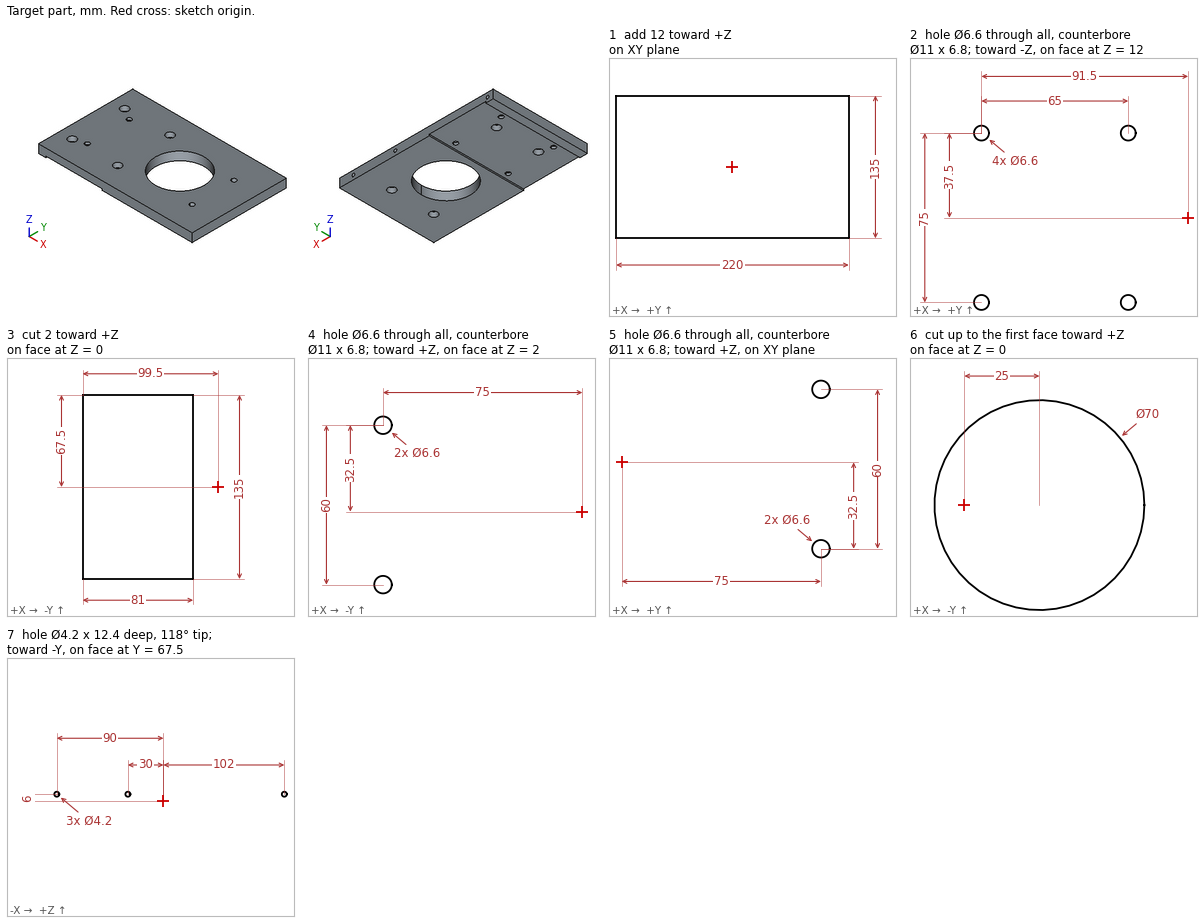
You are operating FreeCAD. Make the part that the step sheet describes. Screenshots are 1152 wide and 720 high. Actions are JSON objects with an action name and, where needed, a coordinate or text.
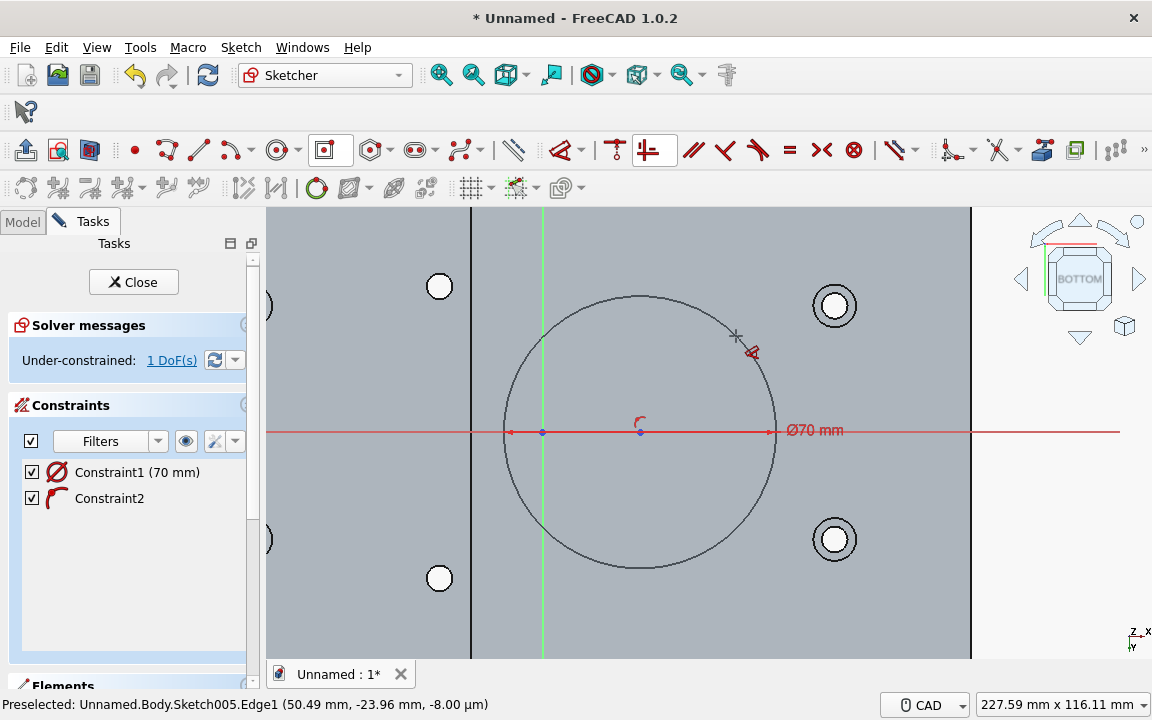
{"action": "left_click", "coordinate": [640, 432]}
{"action": "left_click", "coordinate": [591, 466]}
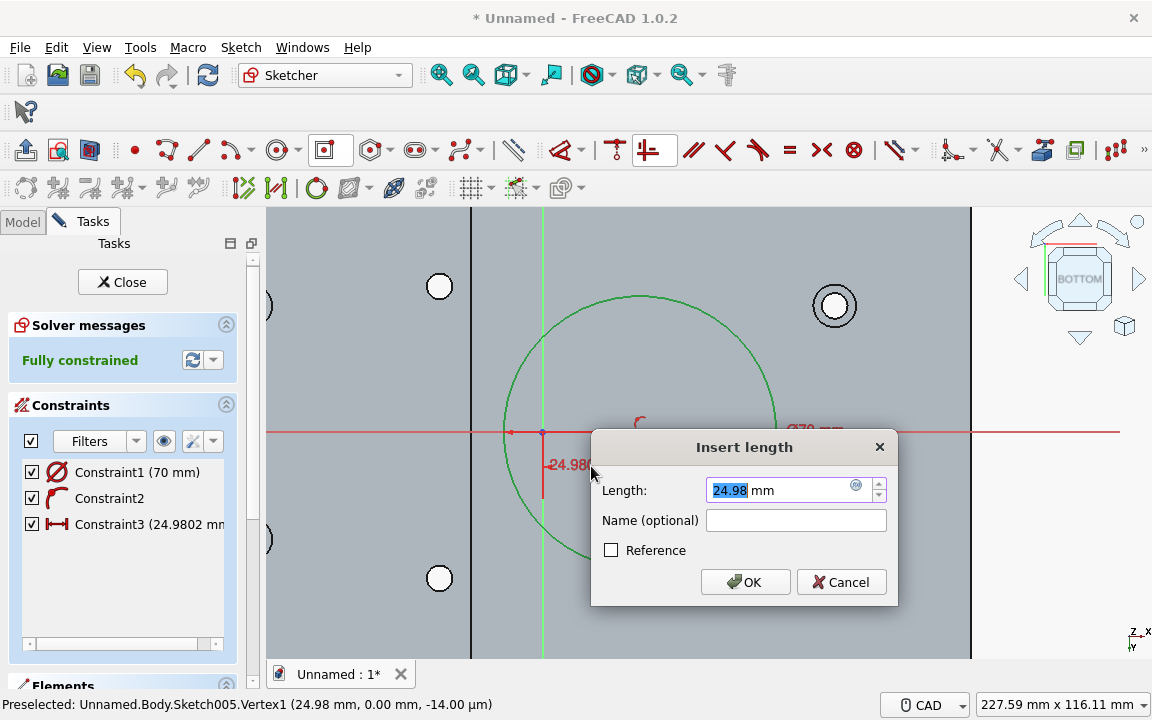
{"action": "type", "text": "25"}
{"action": "key", "text": "Return"}
{"action": "key", "text": "Escape"}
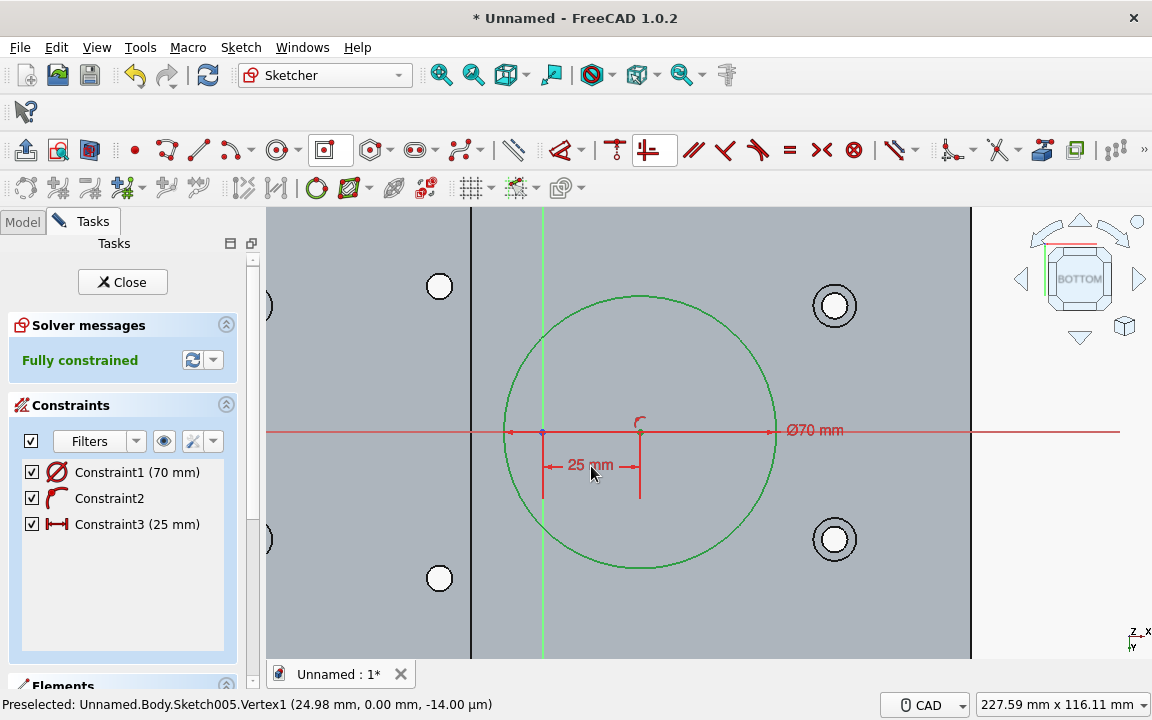
{"action": "left_click", "coordinate": [123, 282]}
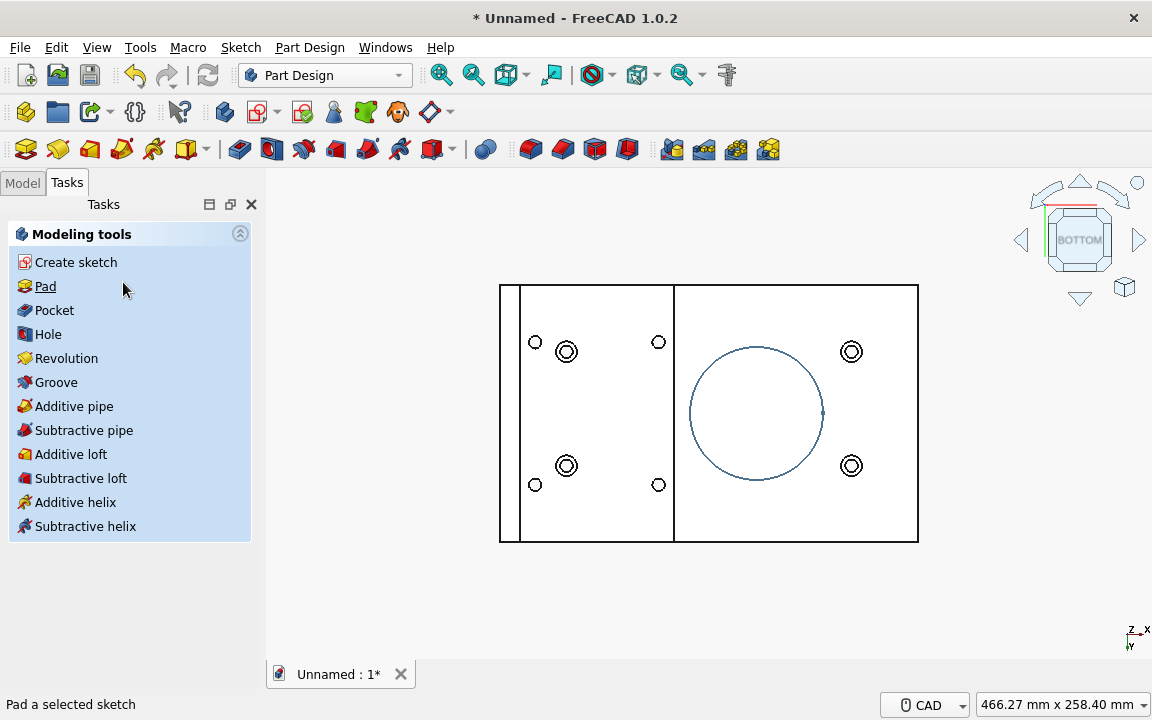
{"action": "left_click", "coordinate": [240, 150]}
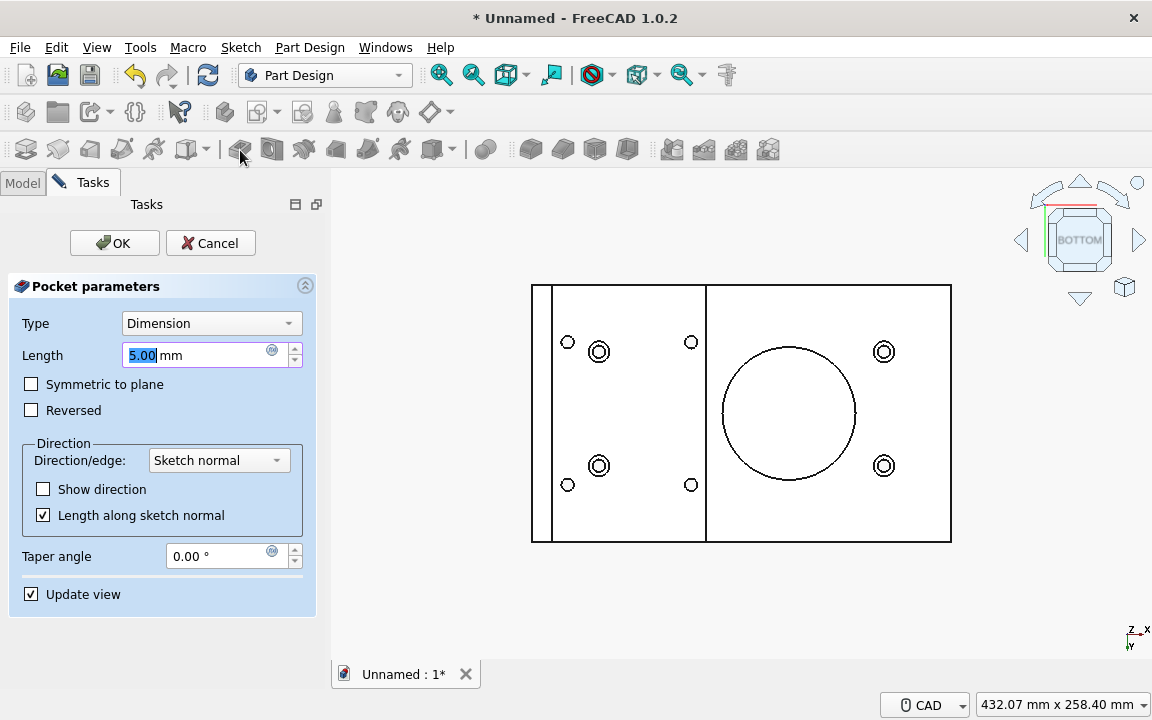
{"action": "left_click", "coordinate": [212, 324]}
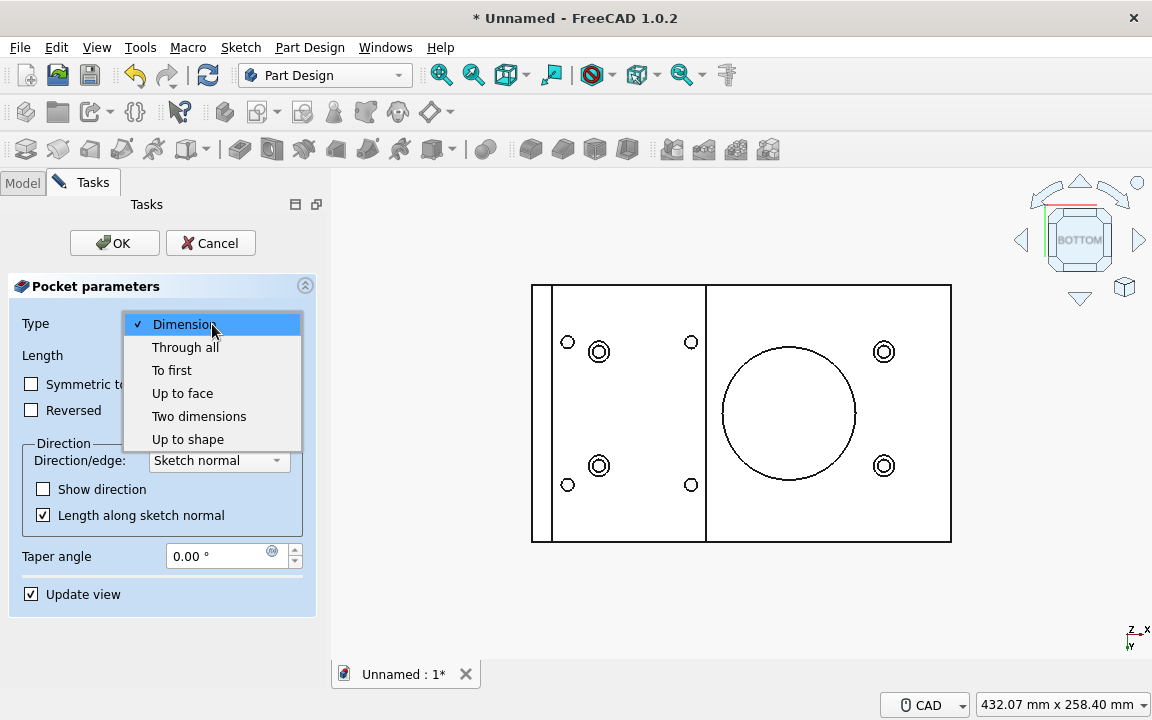
{"action": "left_click", "coordinate": [212, 370]}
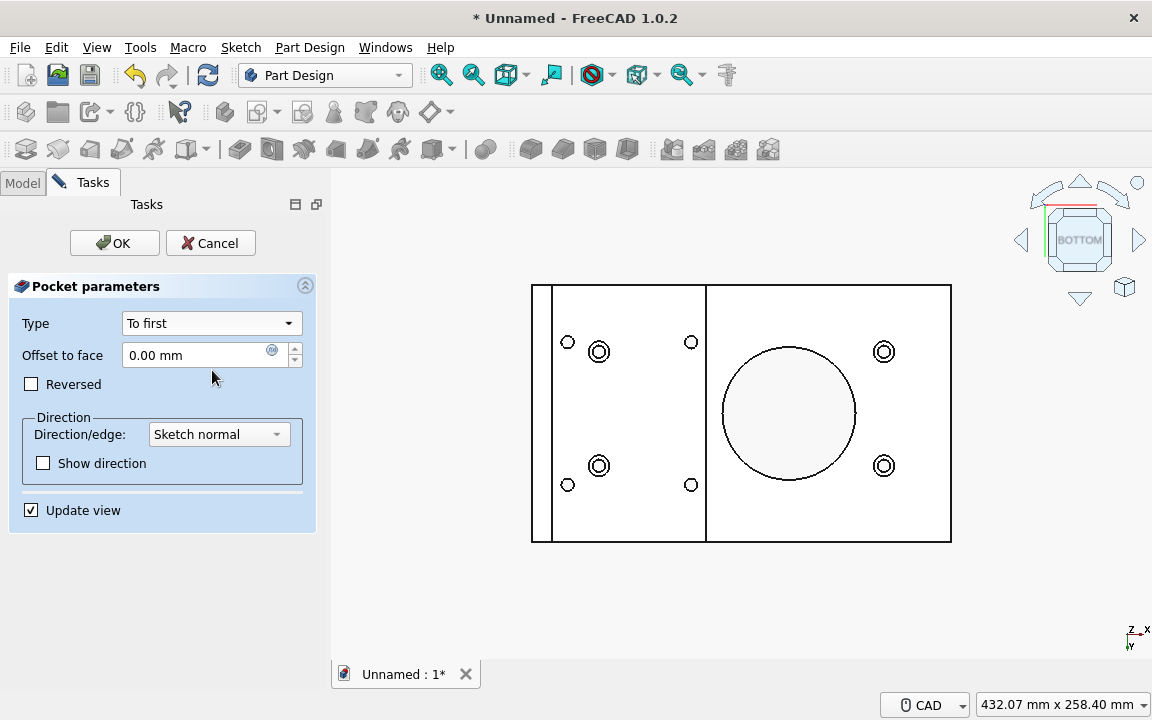
{"action": "left_click", "coordinate": [115, 243]}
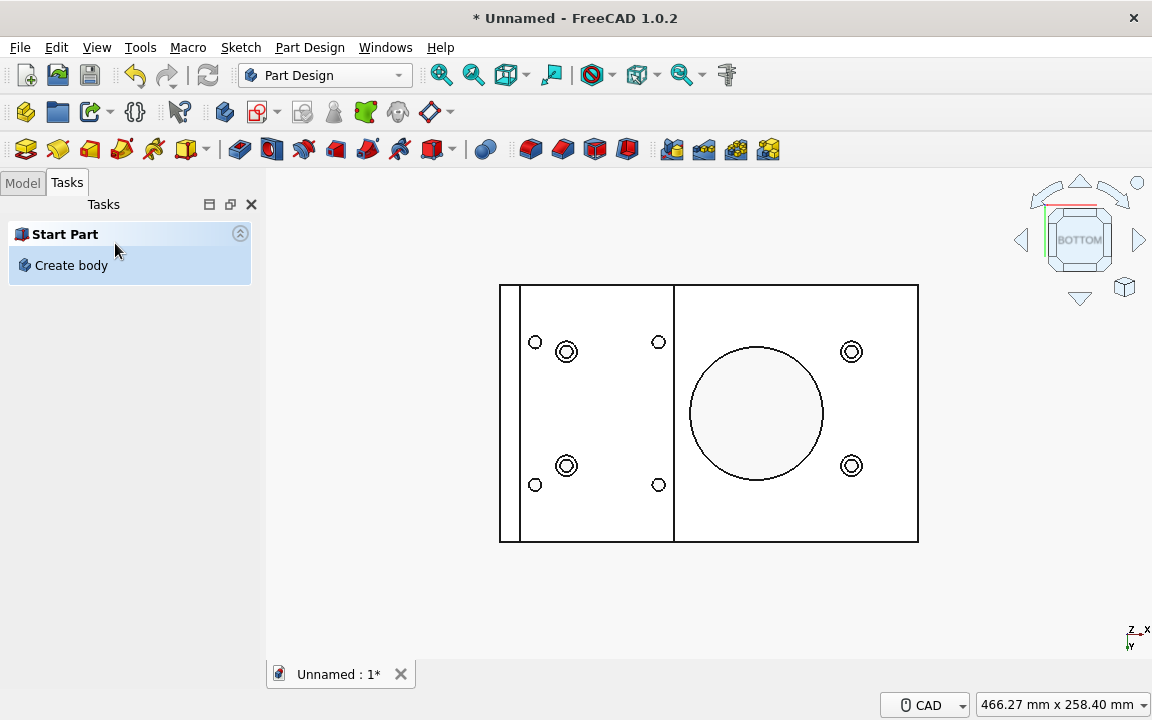
{"action": "key", "text": "4"}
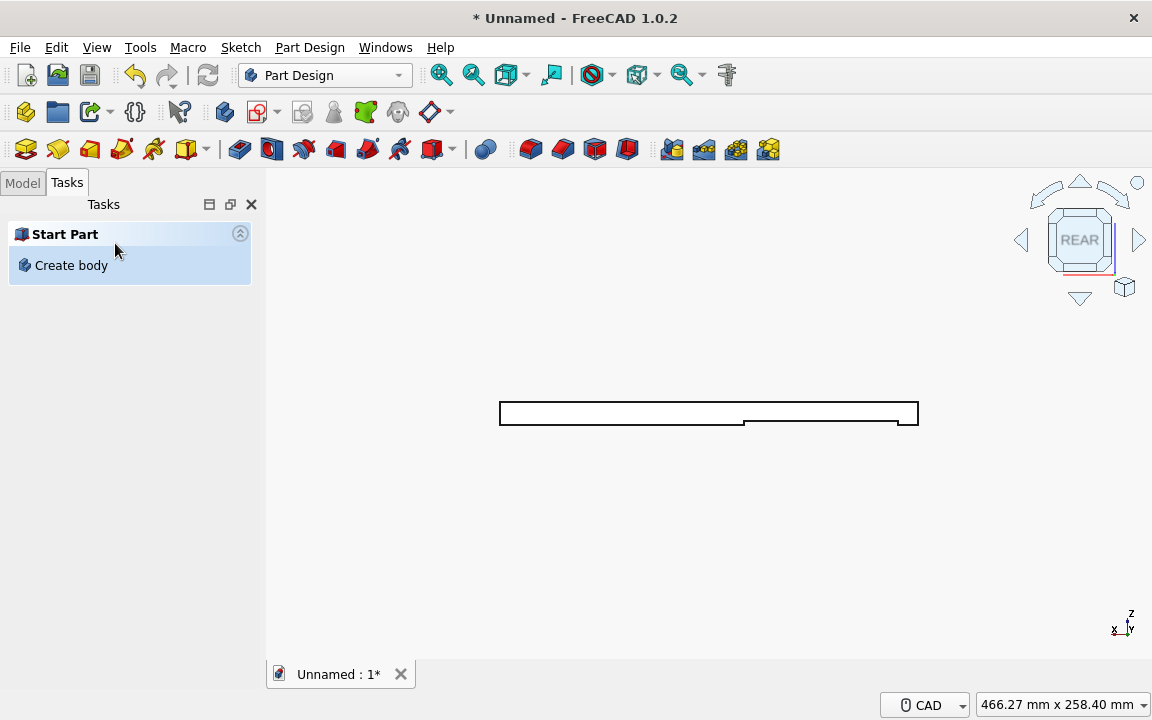
{"action": "left_click", "coordinate": [530, 412]}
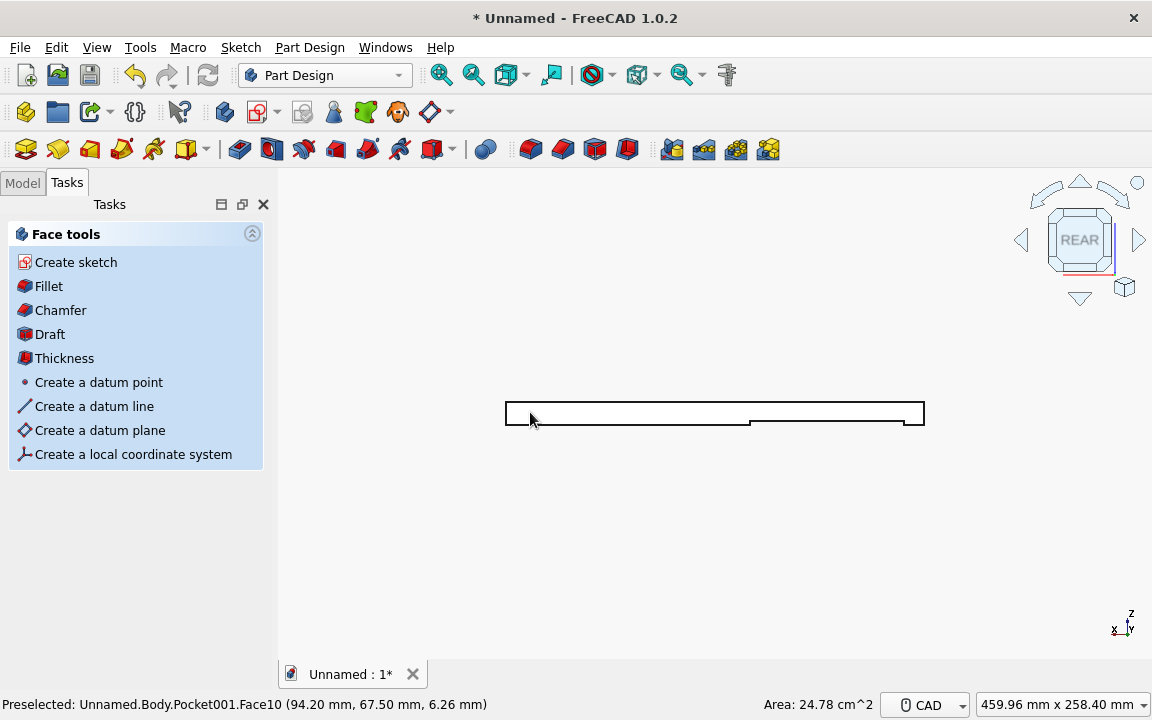
{"action": "left_click", "coordinate": [258, 112]}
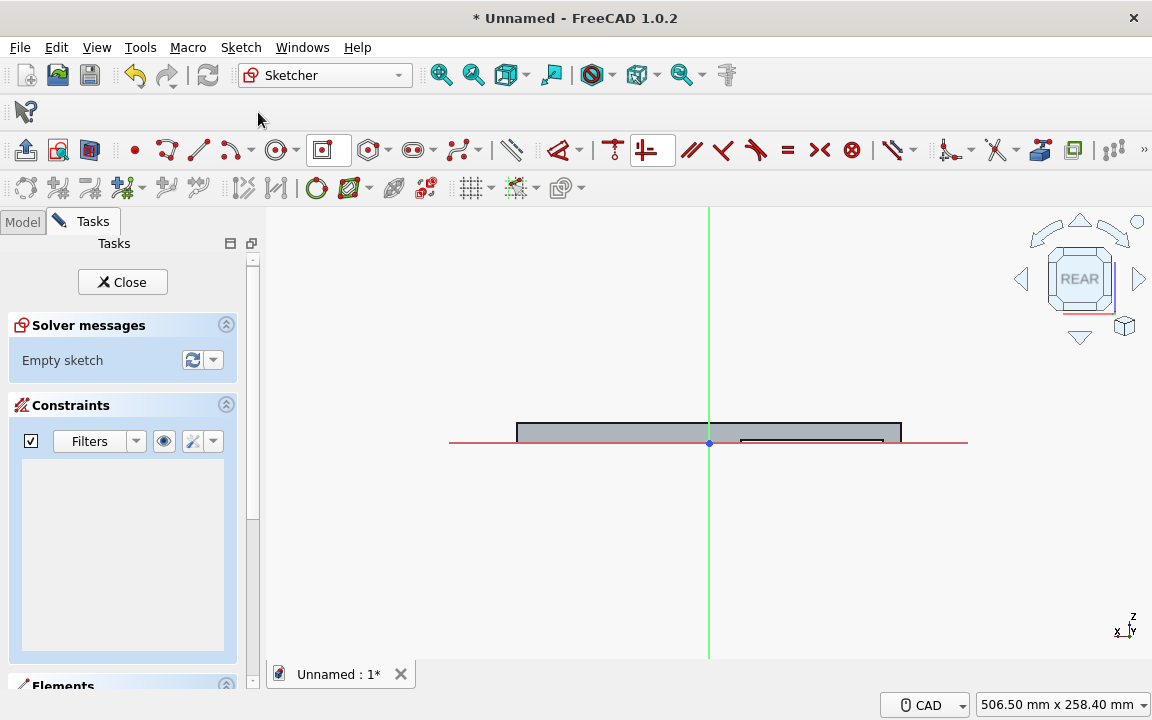
{"action": "scroll", "coordinate": [880, 443], "scroll_direction": "up", "scroll_amount": 2}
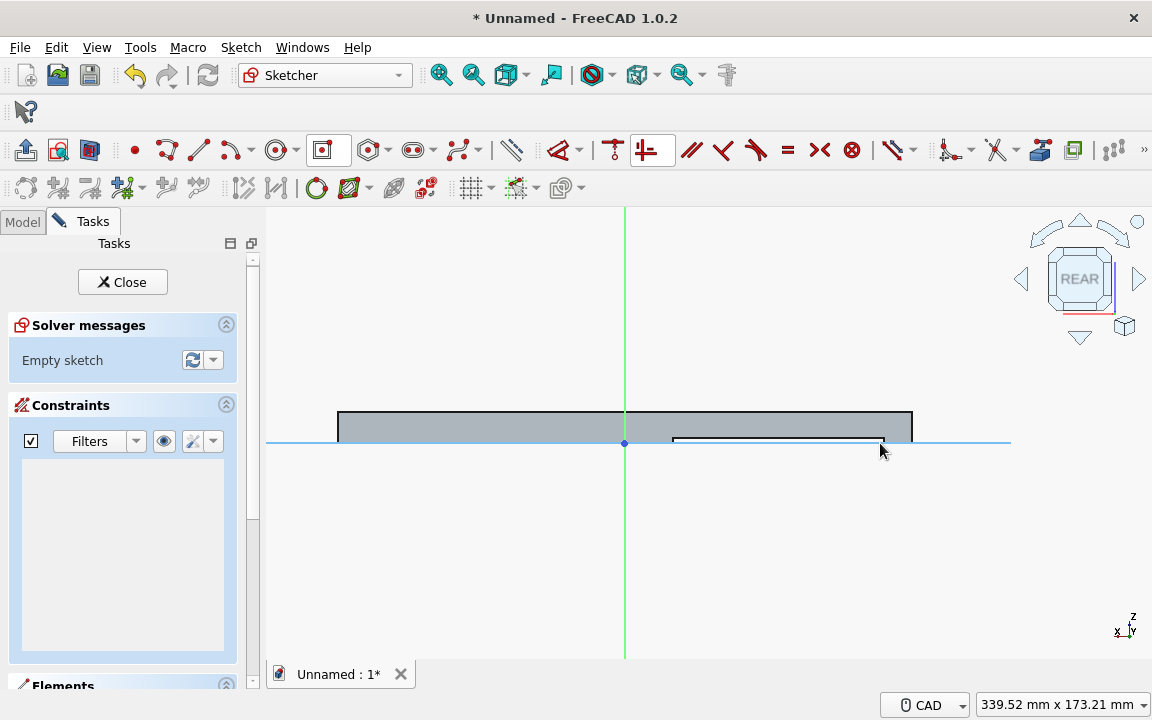
{"action": "left_click", "coordinate": [276, 150]}